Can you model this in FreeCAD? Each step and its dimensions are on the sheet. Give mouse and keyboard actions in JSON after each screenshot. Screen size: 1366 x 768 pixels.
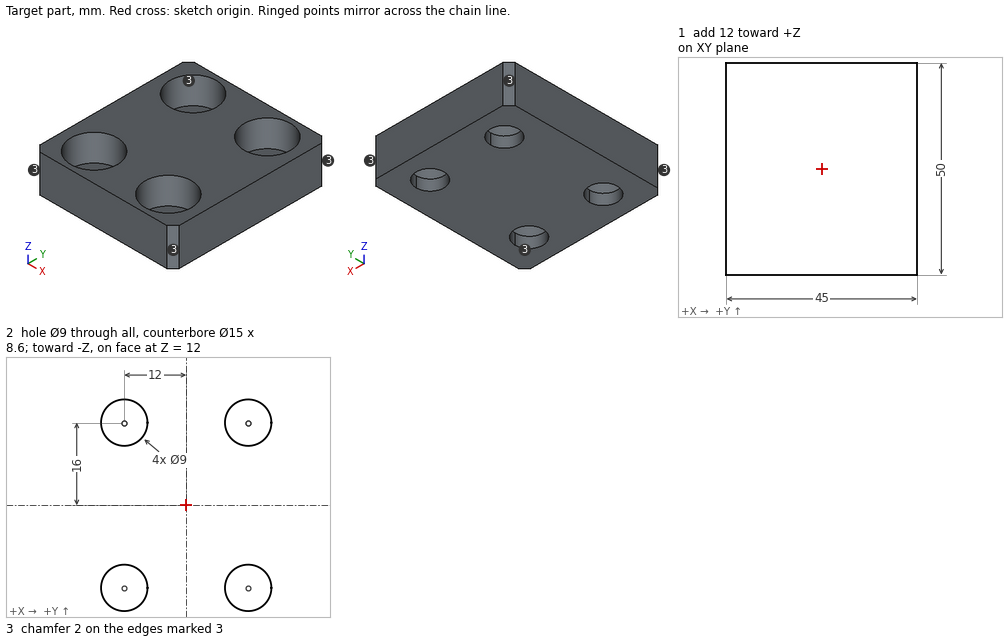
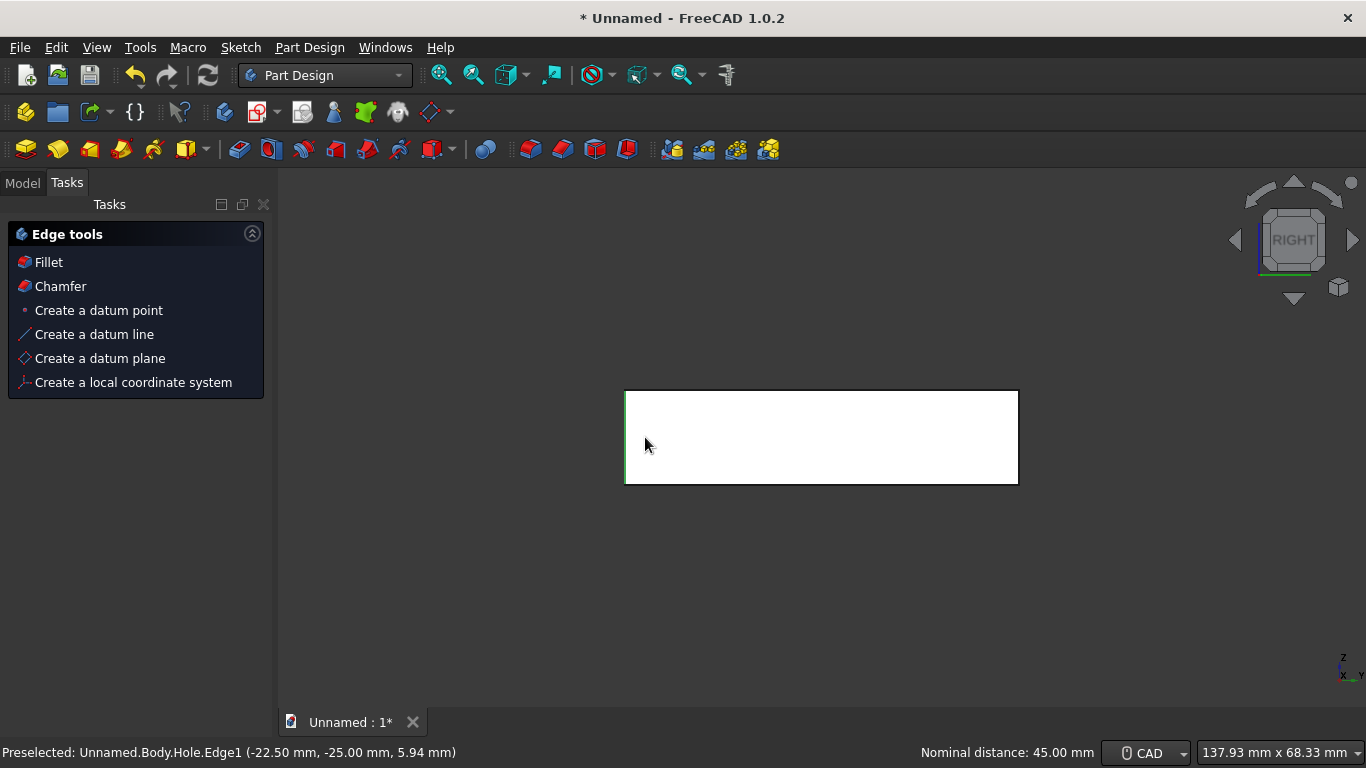
{"action": "left_click", "coordinate": [442, 76]}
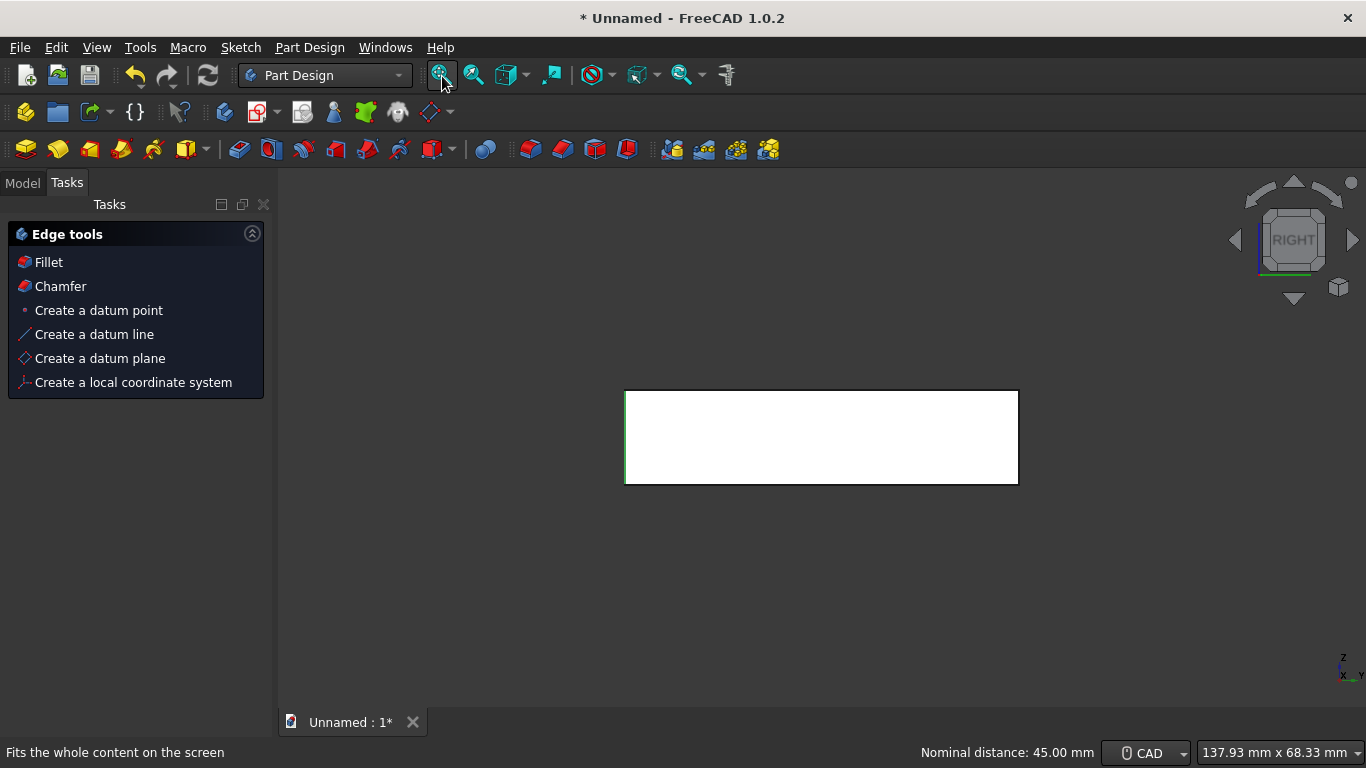
{"action": "left_click", "coordinate": [1019, 436], "text": "ctrl"}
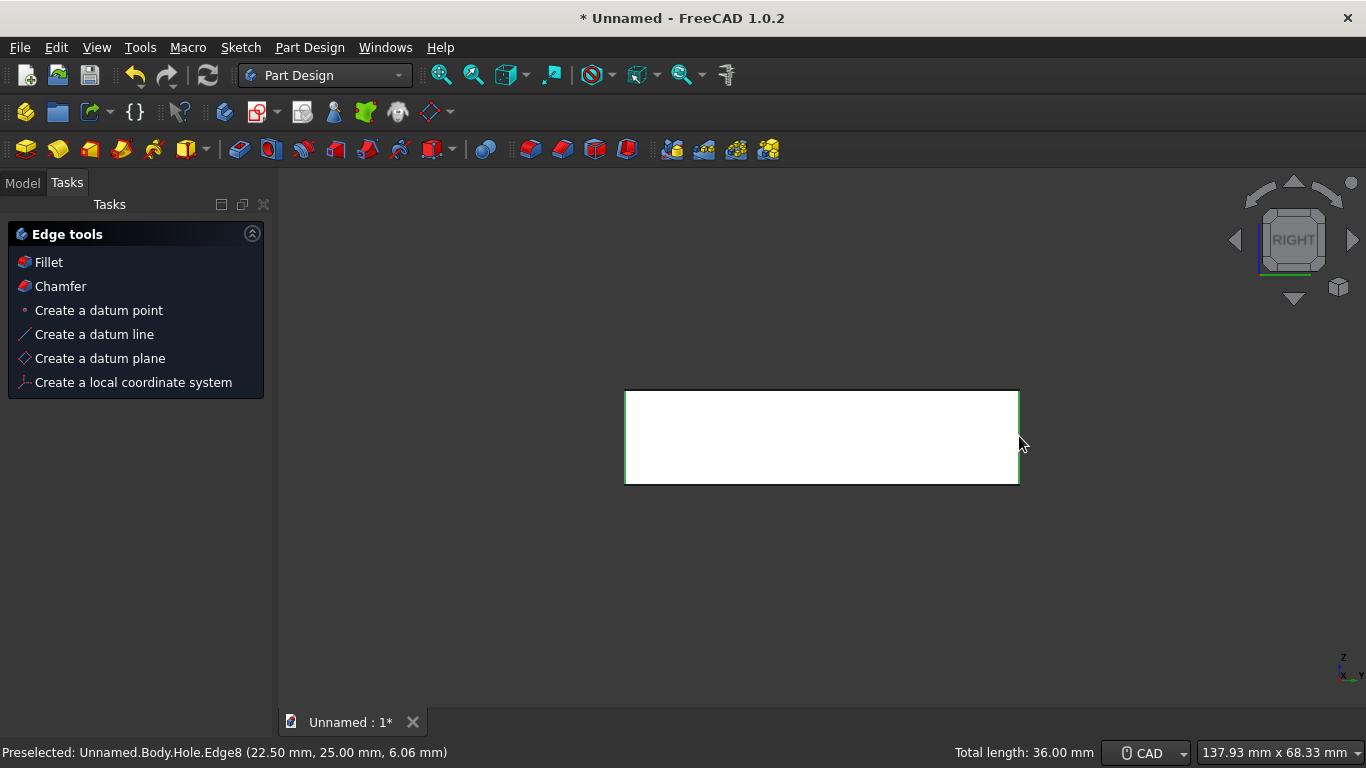
{"action": "key", "text": "5"}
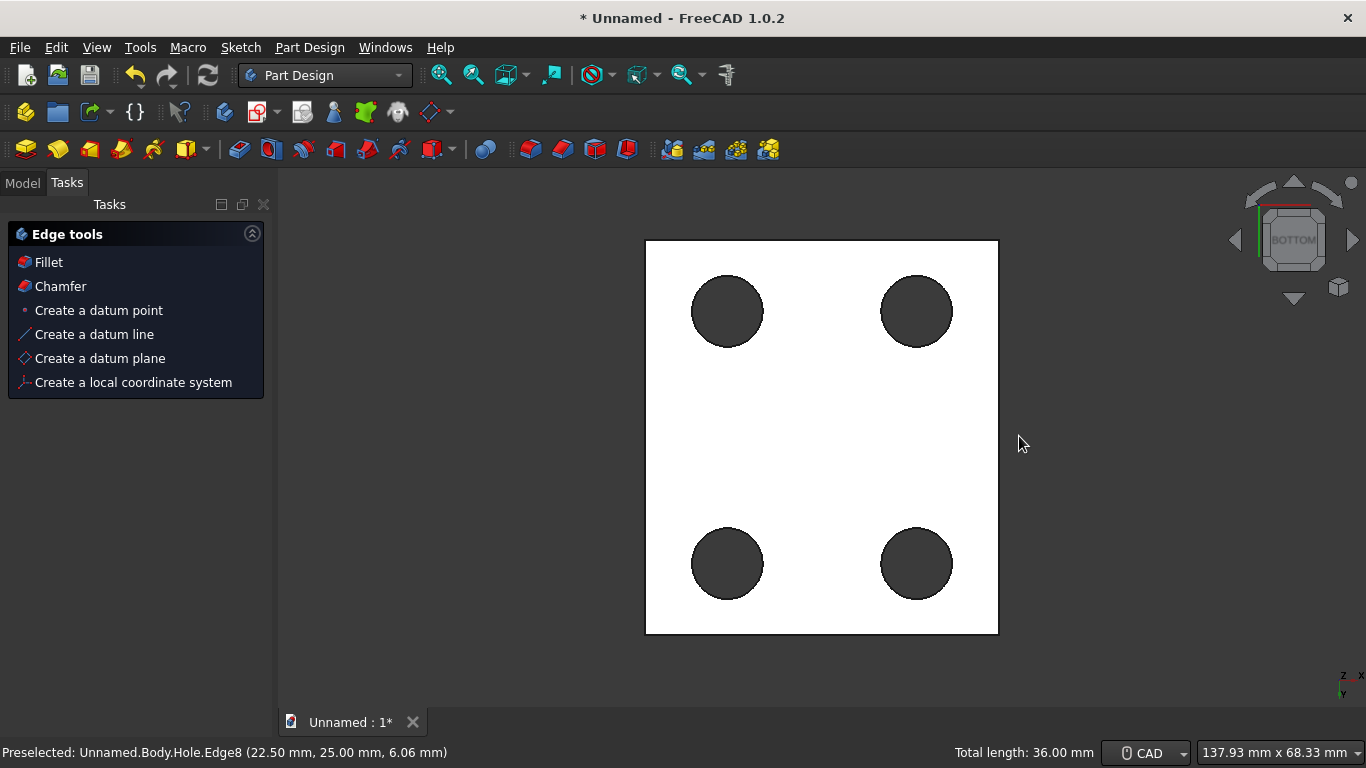
{"action": "key", "text": "4"}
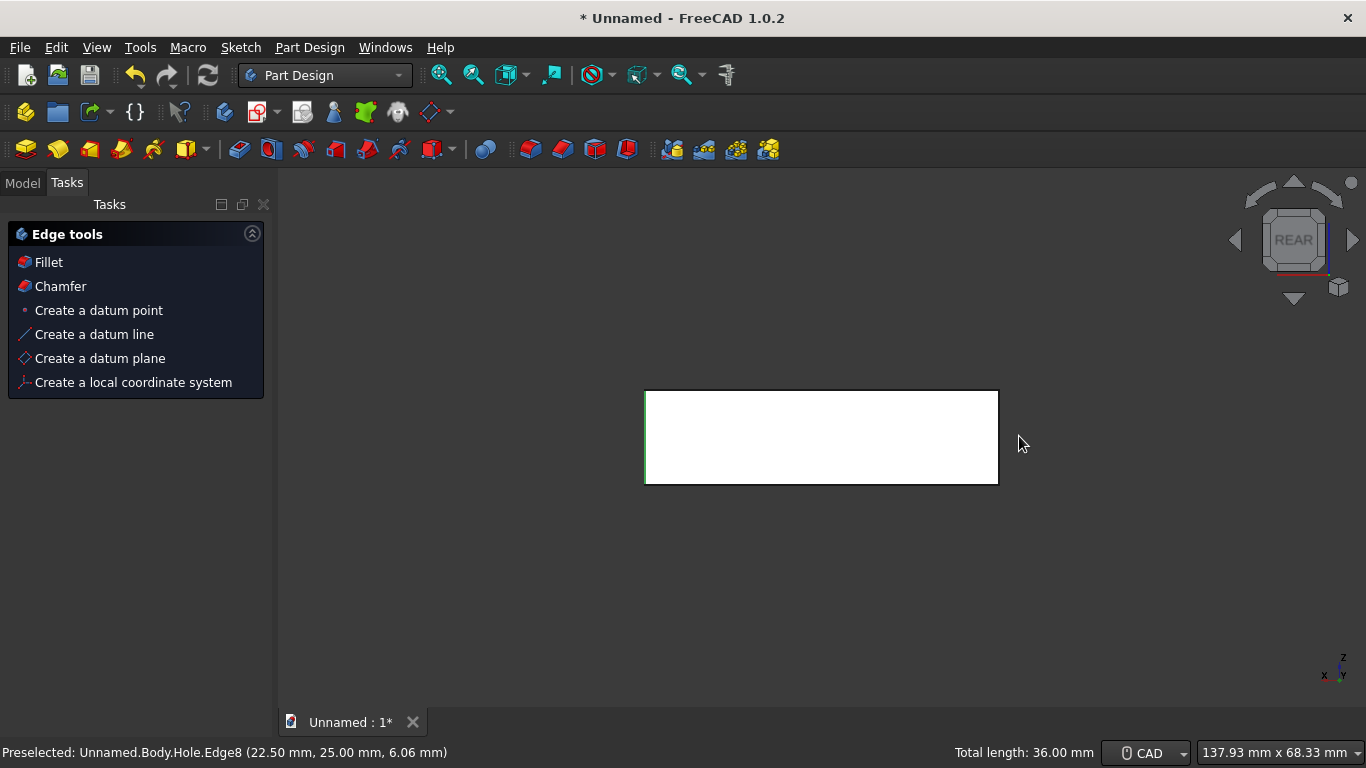
{"action": "left_click", "coordinate": [442, 76]}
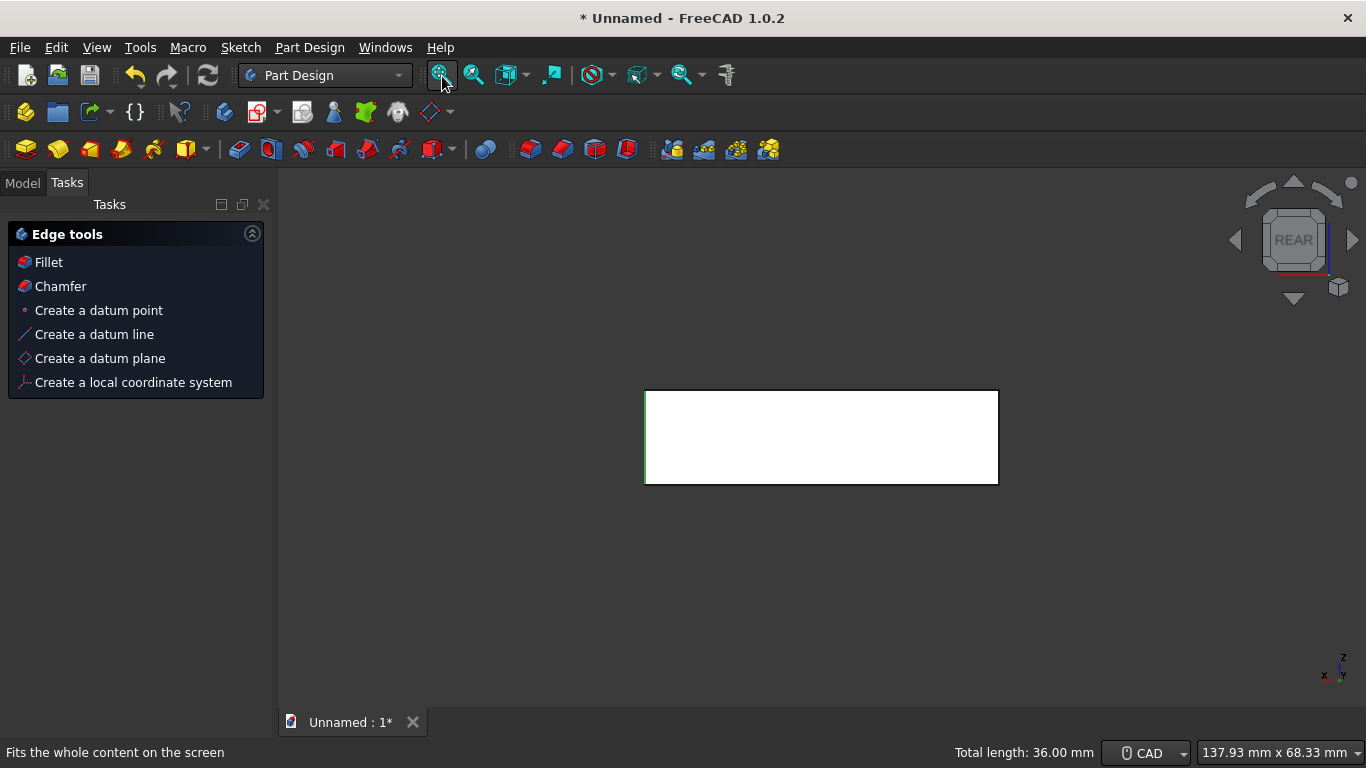
{"action": "left_click", "coordinate": [999, 437], "text": "ctrl"}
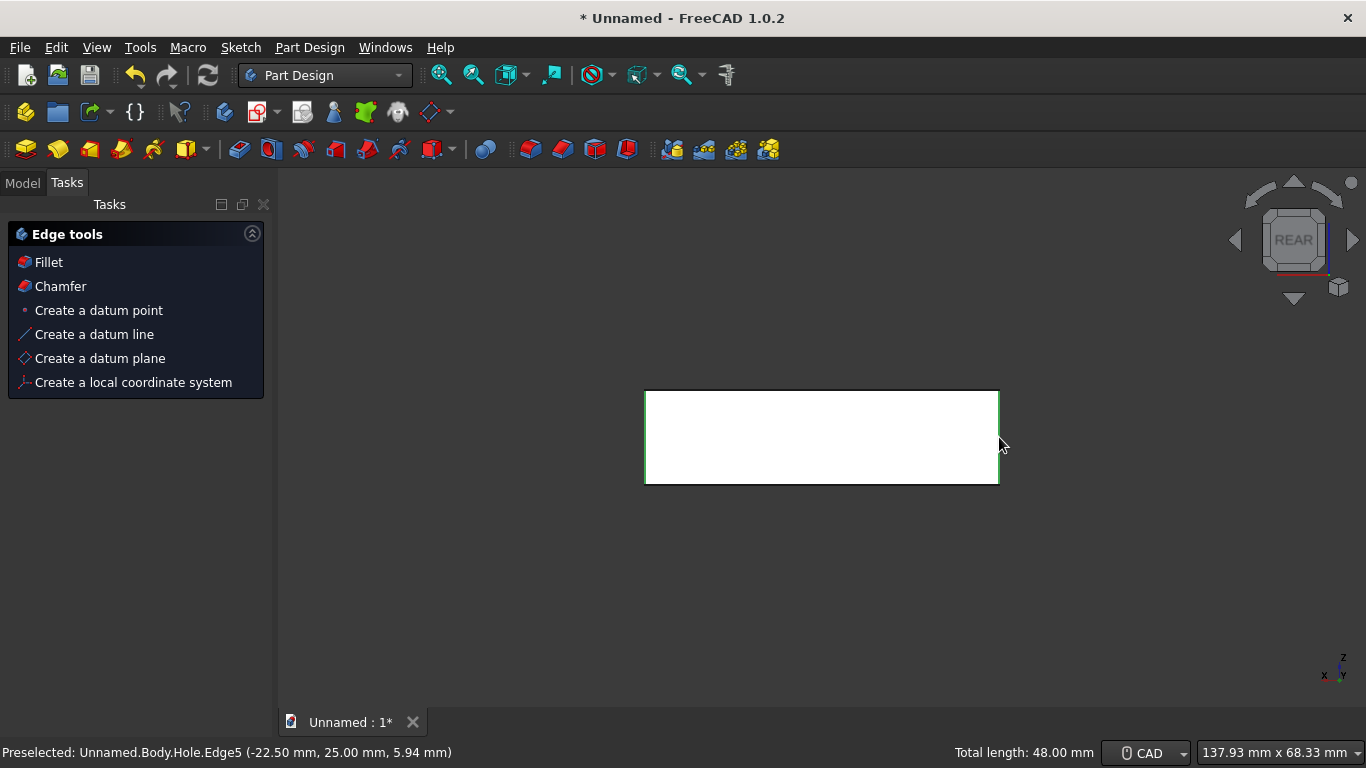
{"action": "left_click", "coordinate": [564, 150]}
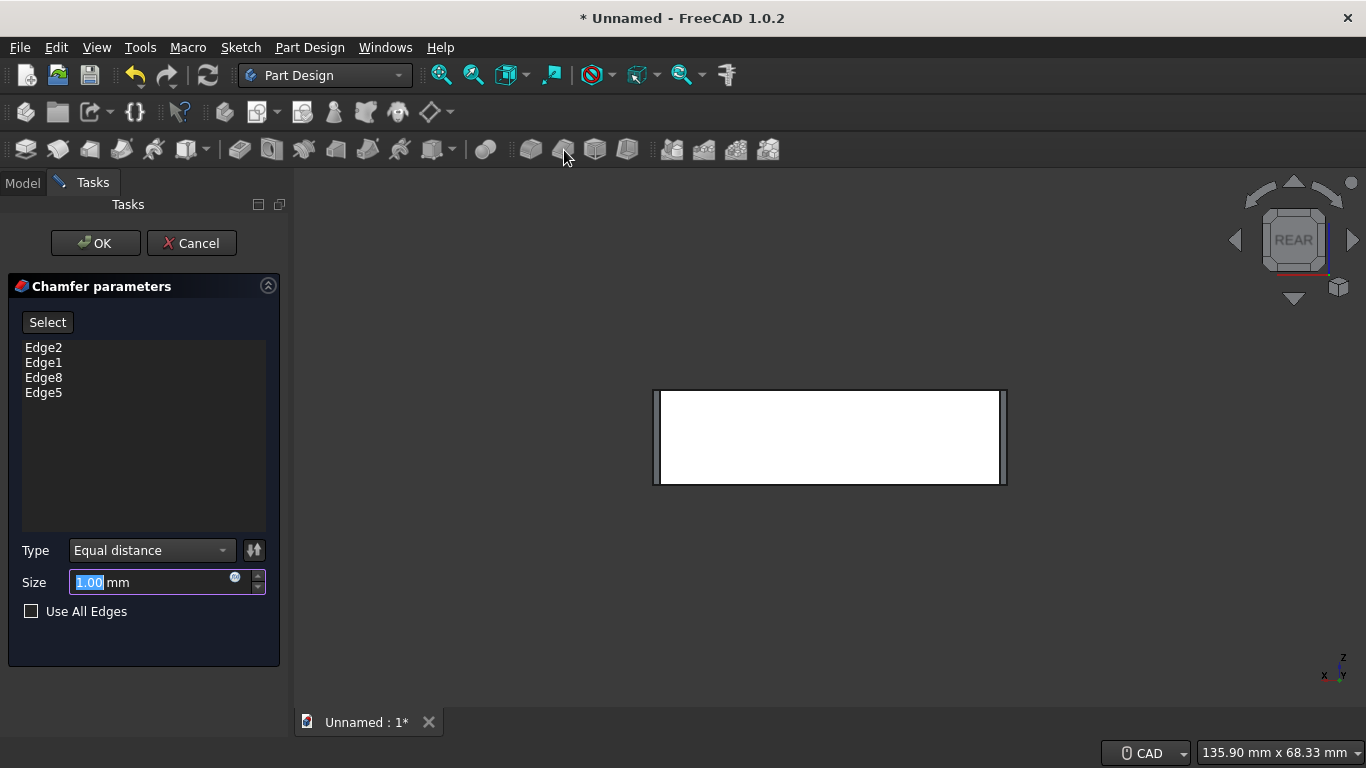
{"action": "type", "text": "2"}
{"action": "key", "text": "Tab"}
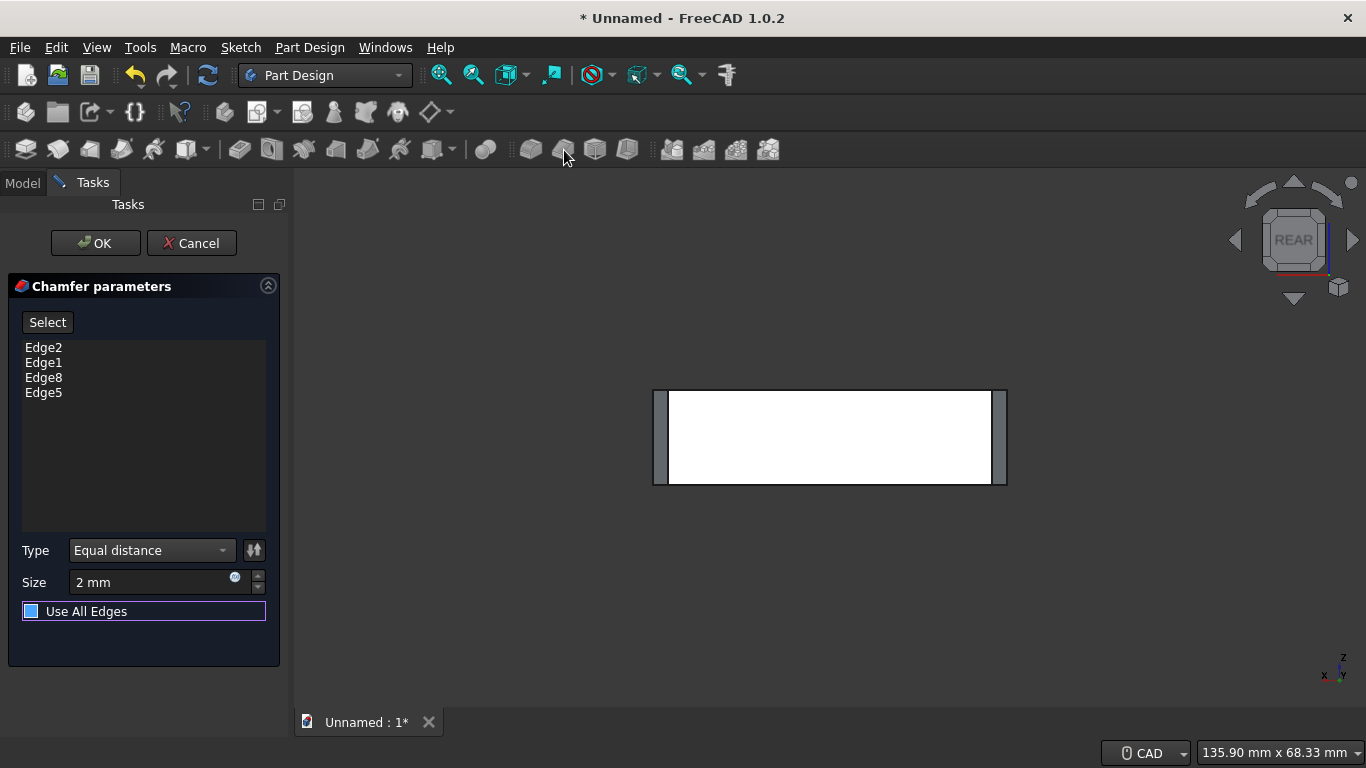
{"action": "left_click", "coordinate": [96, 243]}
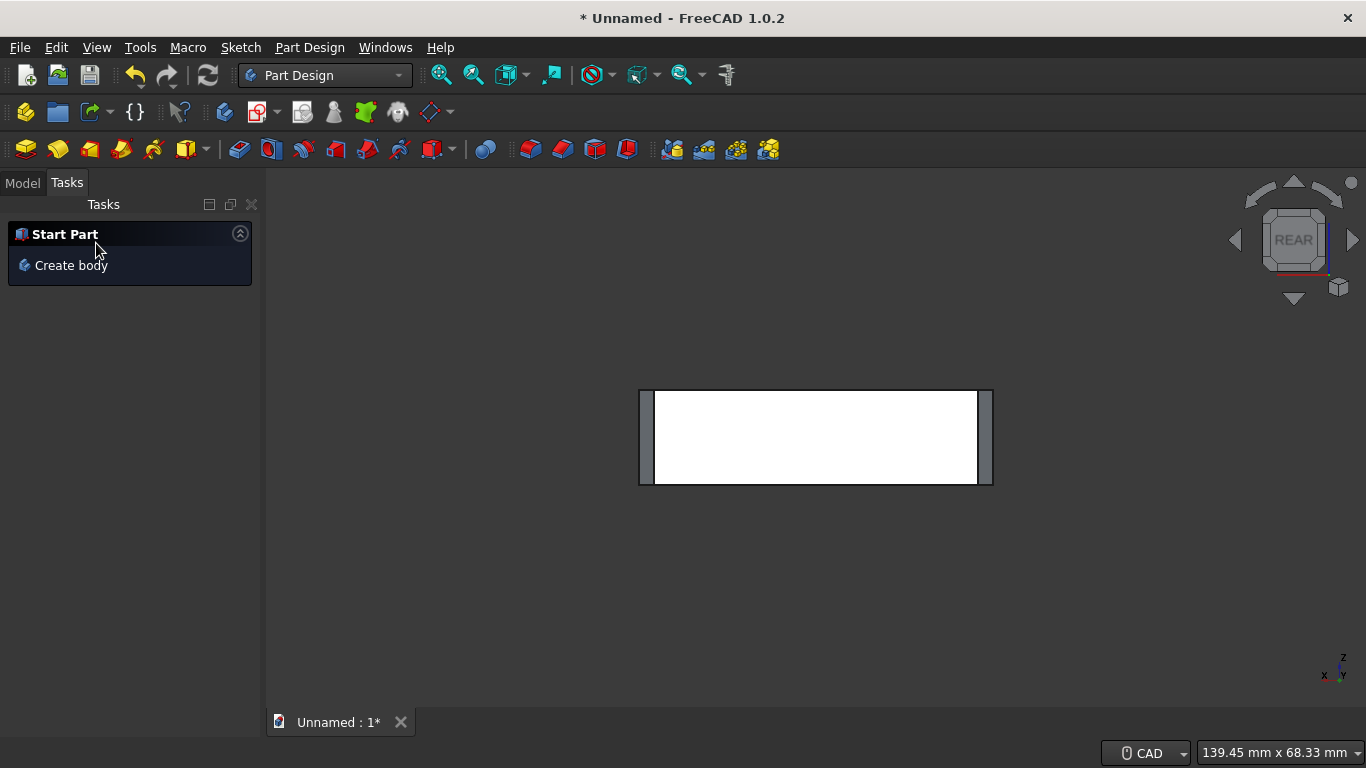
{"action": "key", "text": "0"}